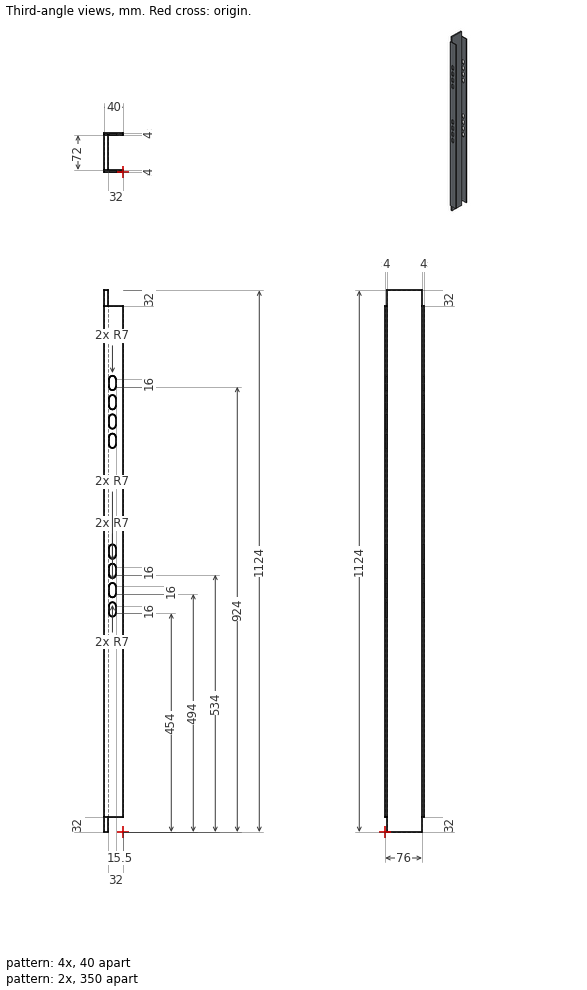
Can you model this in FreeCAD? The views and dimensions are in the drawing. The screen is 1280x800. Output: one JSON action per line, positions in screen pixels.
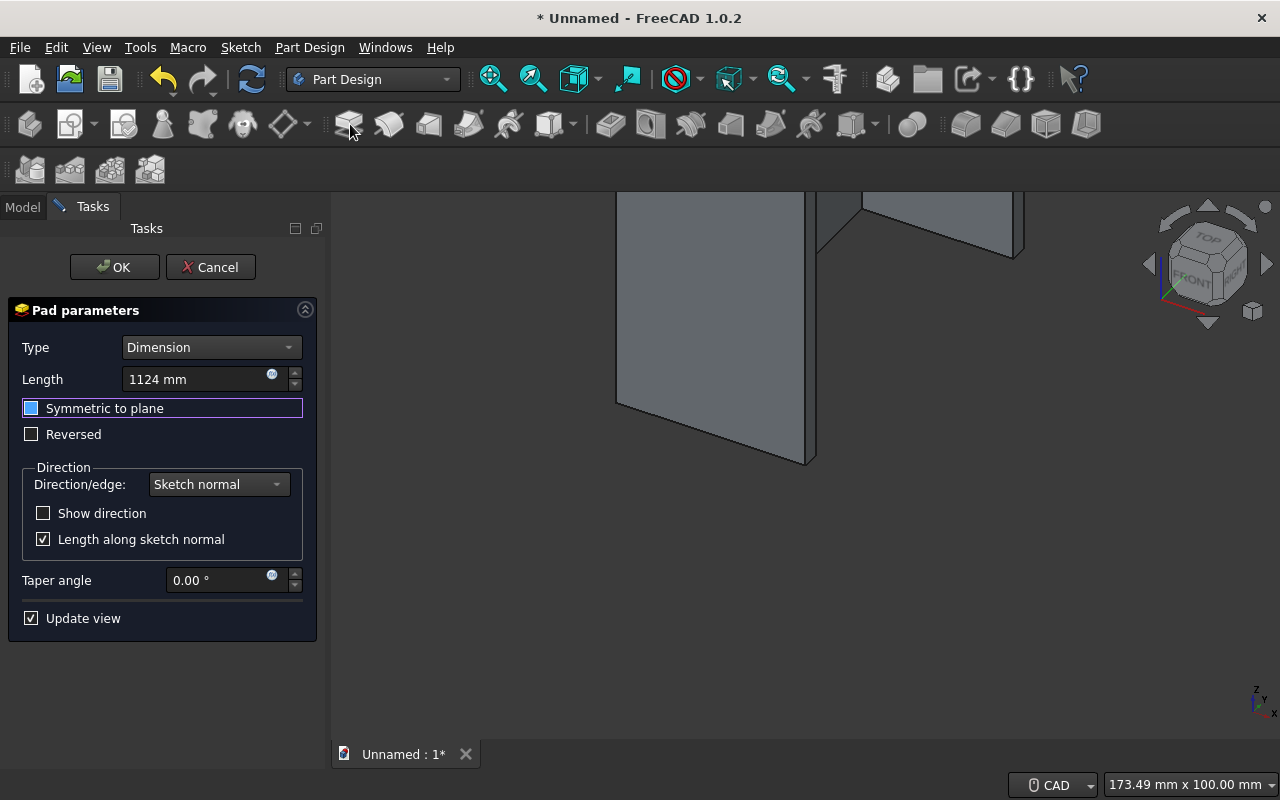
{"action": "left_click", "coordinate": [115, 267]}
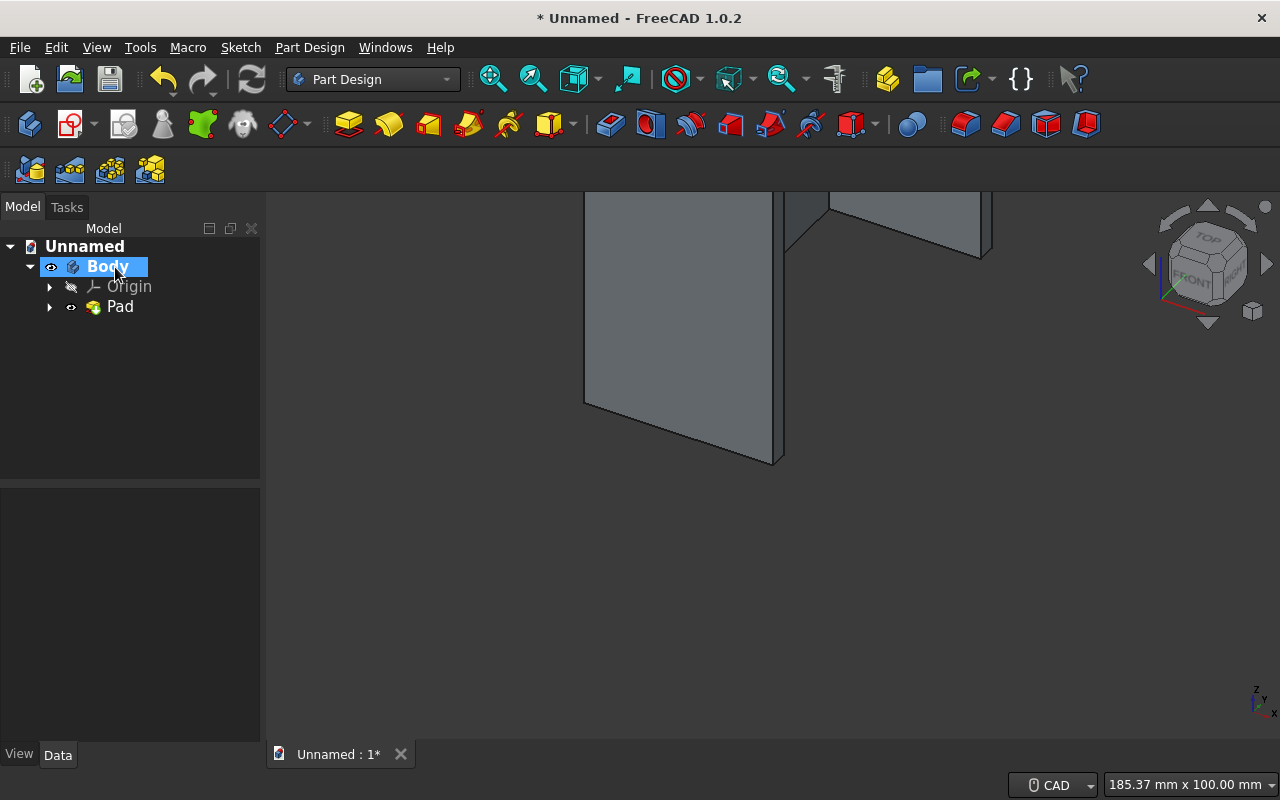
{"action": "key", "text": "v f"}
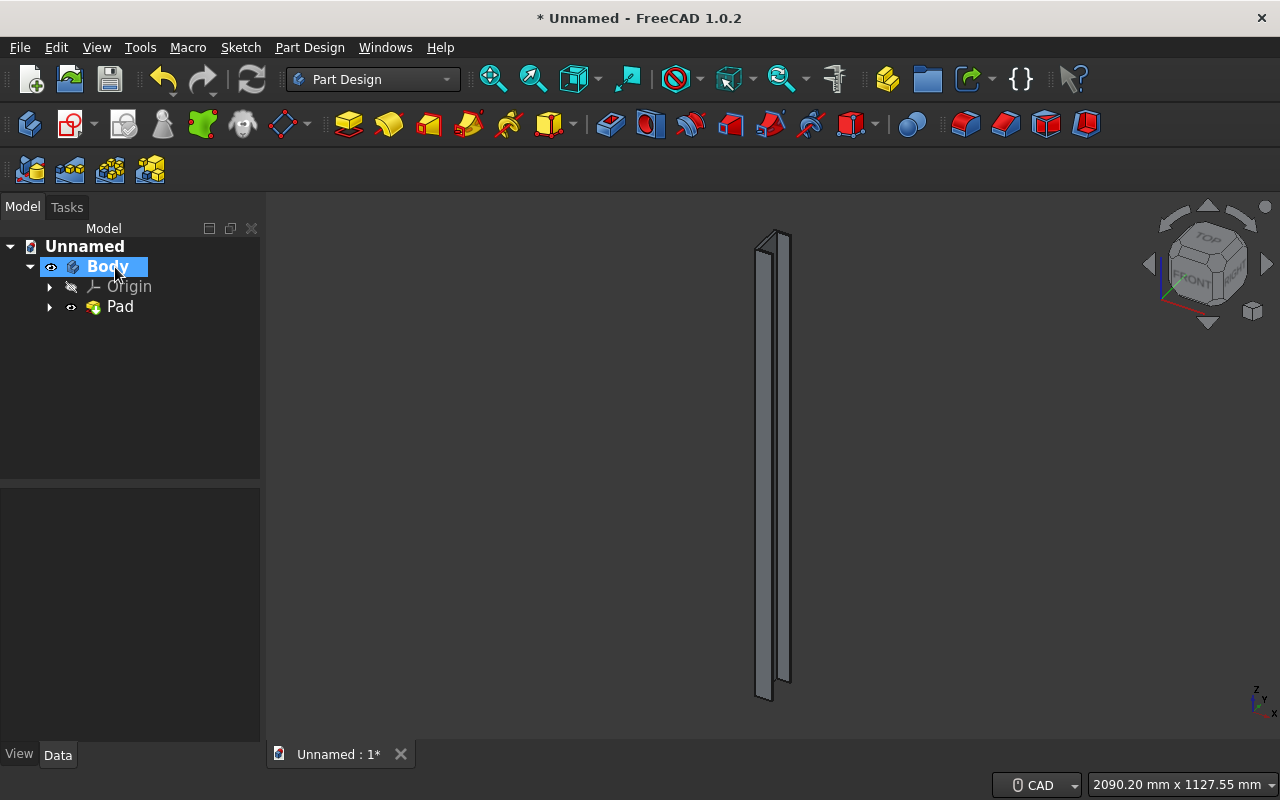
{"action": "key", "text": "4"}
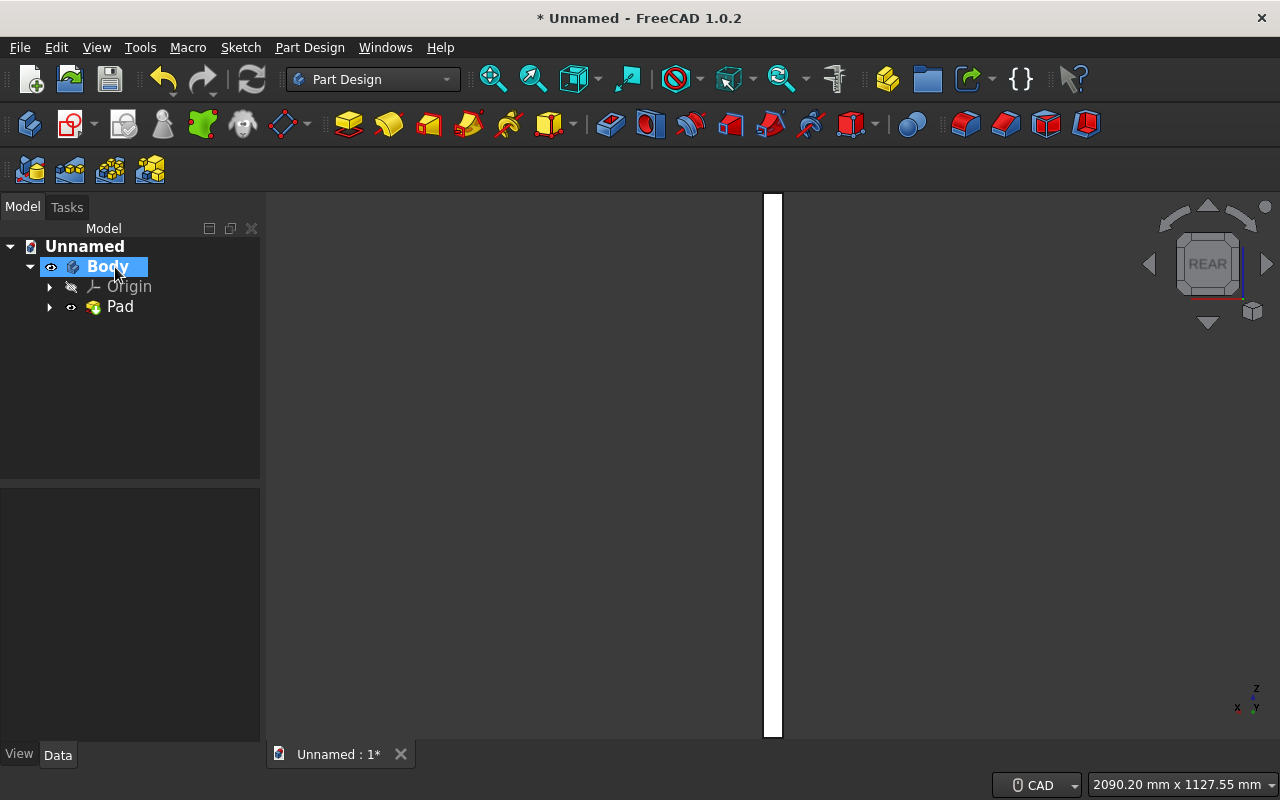
{"action": "left_click", "coordinate": [773, 231]}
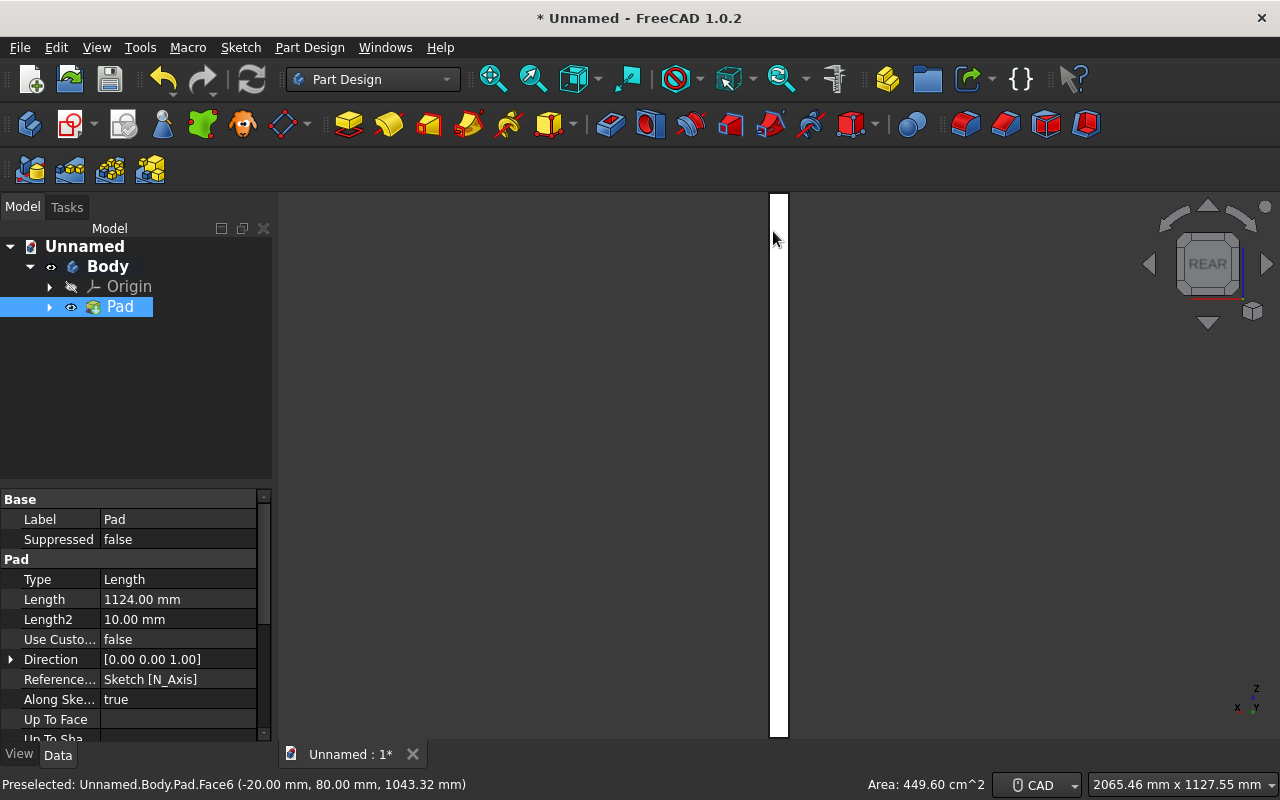
{"action": "left_click", "coordinate": [70, 124]}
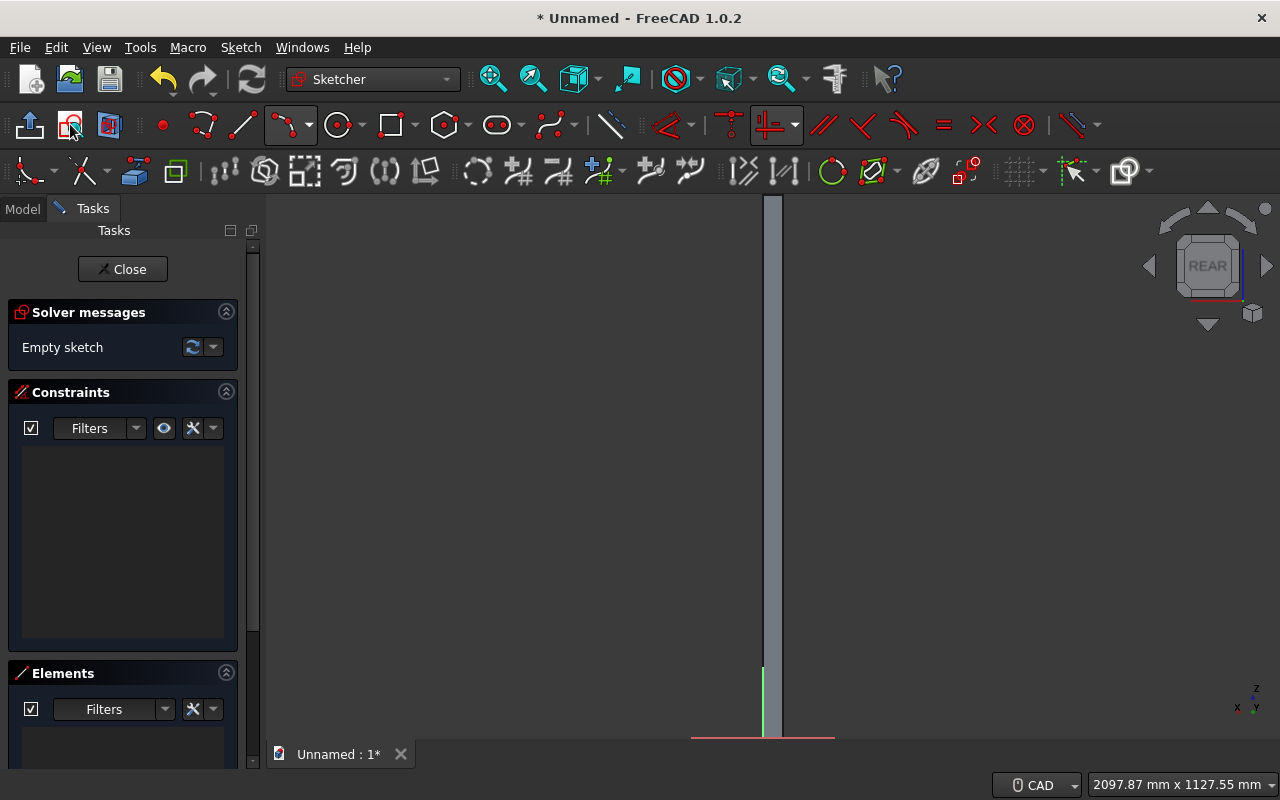
{"action": "scroll", "coordinate": [569, 467], "scroll_direction": "down", "scroll_amount": 2}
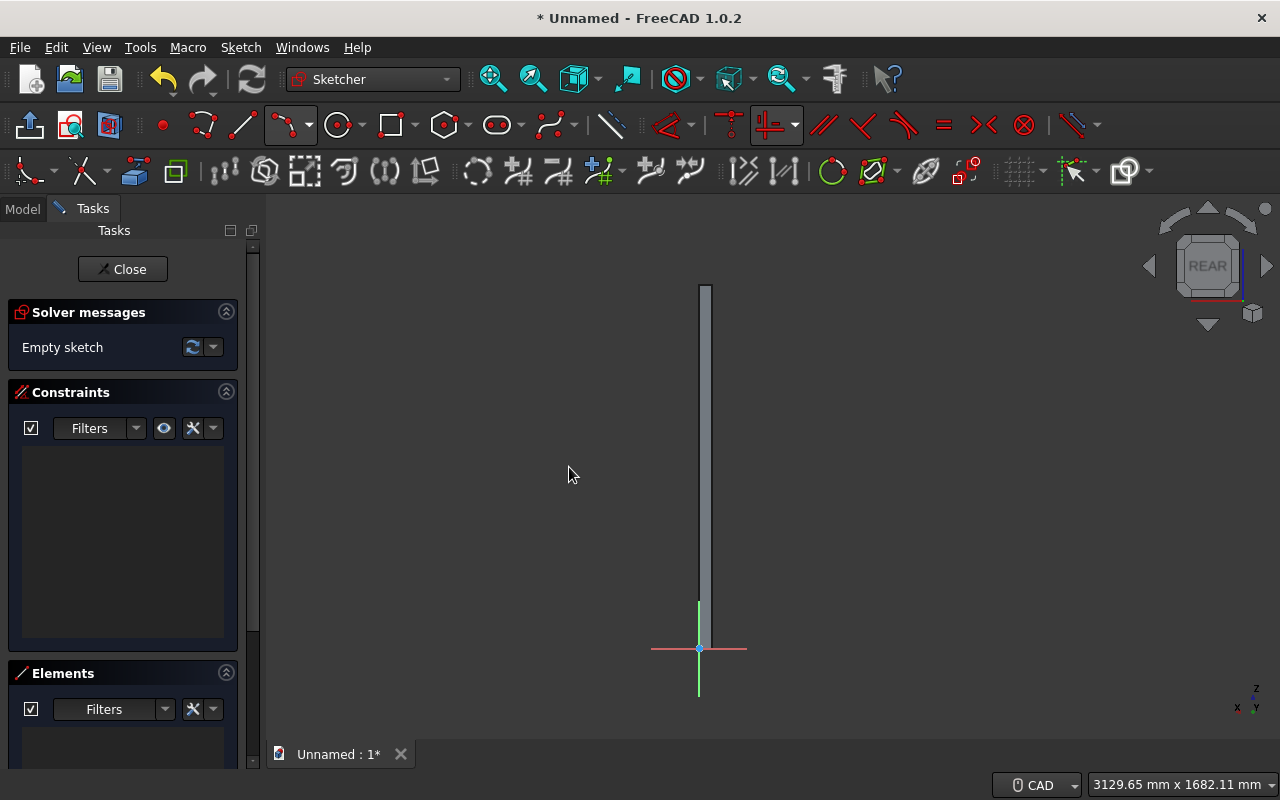
{"action": "left_click", "coordinate": [392, 126]}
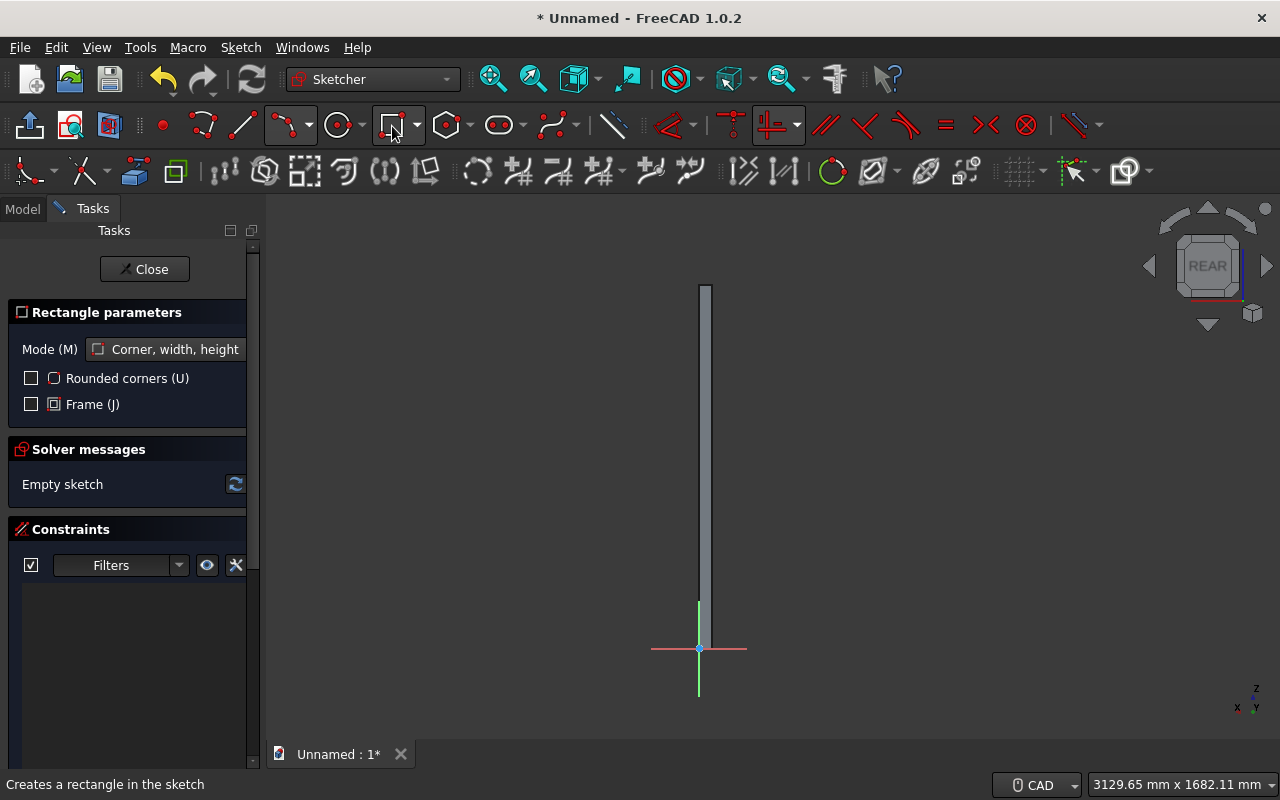
{"action": "scroll", "coordinate": [699, 649], "scroll_direction": "up", "scroll_amount": 3}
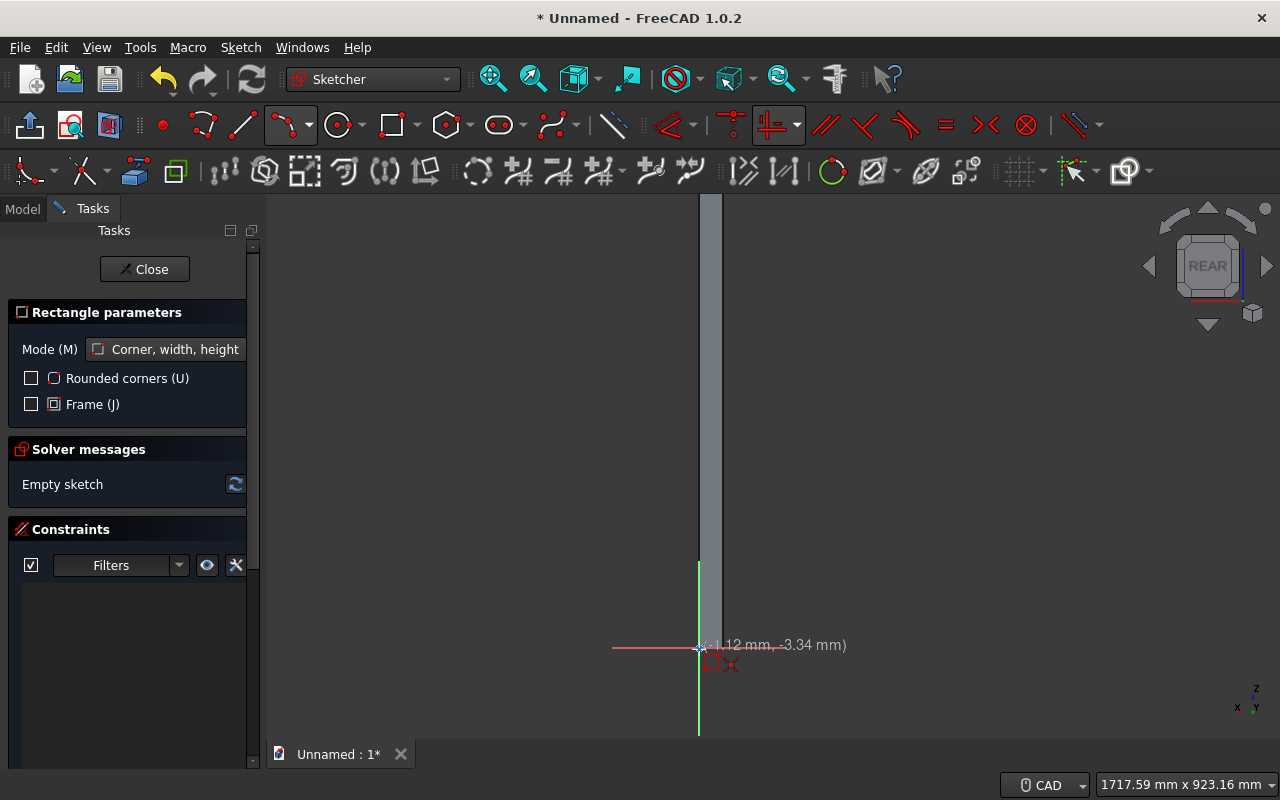
{"action": "left_click", "coordinate": [699, 648]}
{"action": "left_click", "coordinate": [718, 629]}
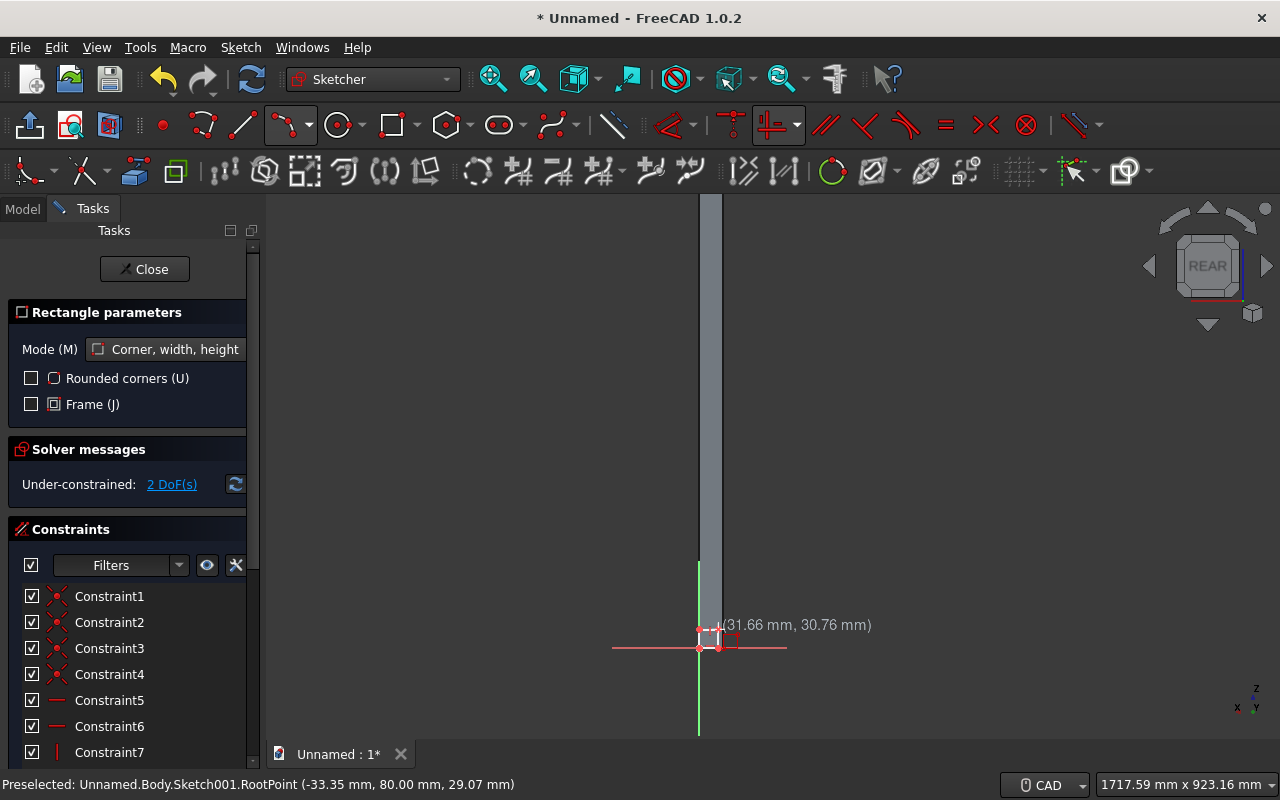
{"action": "scroll", "coordinate": [699, 649], "scroll_direction": "down", "scroll_amount": 3}